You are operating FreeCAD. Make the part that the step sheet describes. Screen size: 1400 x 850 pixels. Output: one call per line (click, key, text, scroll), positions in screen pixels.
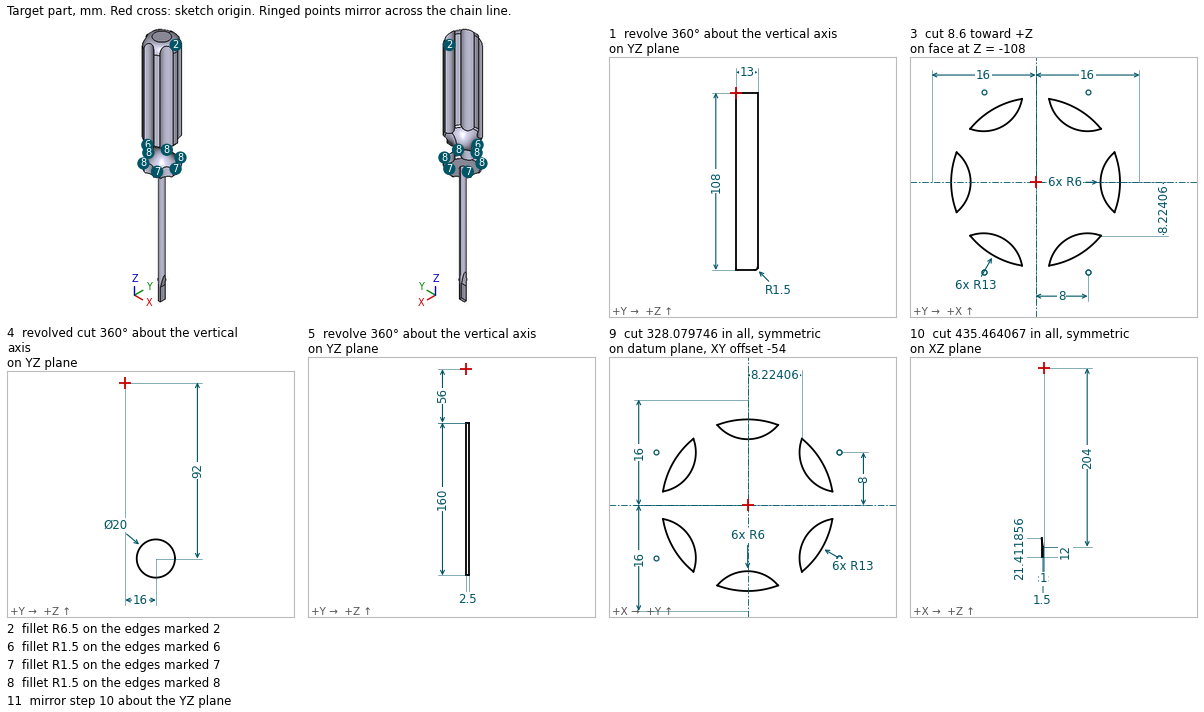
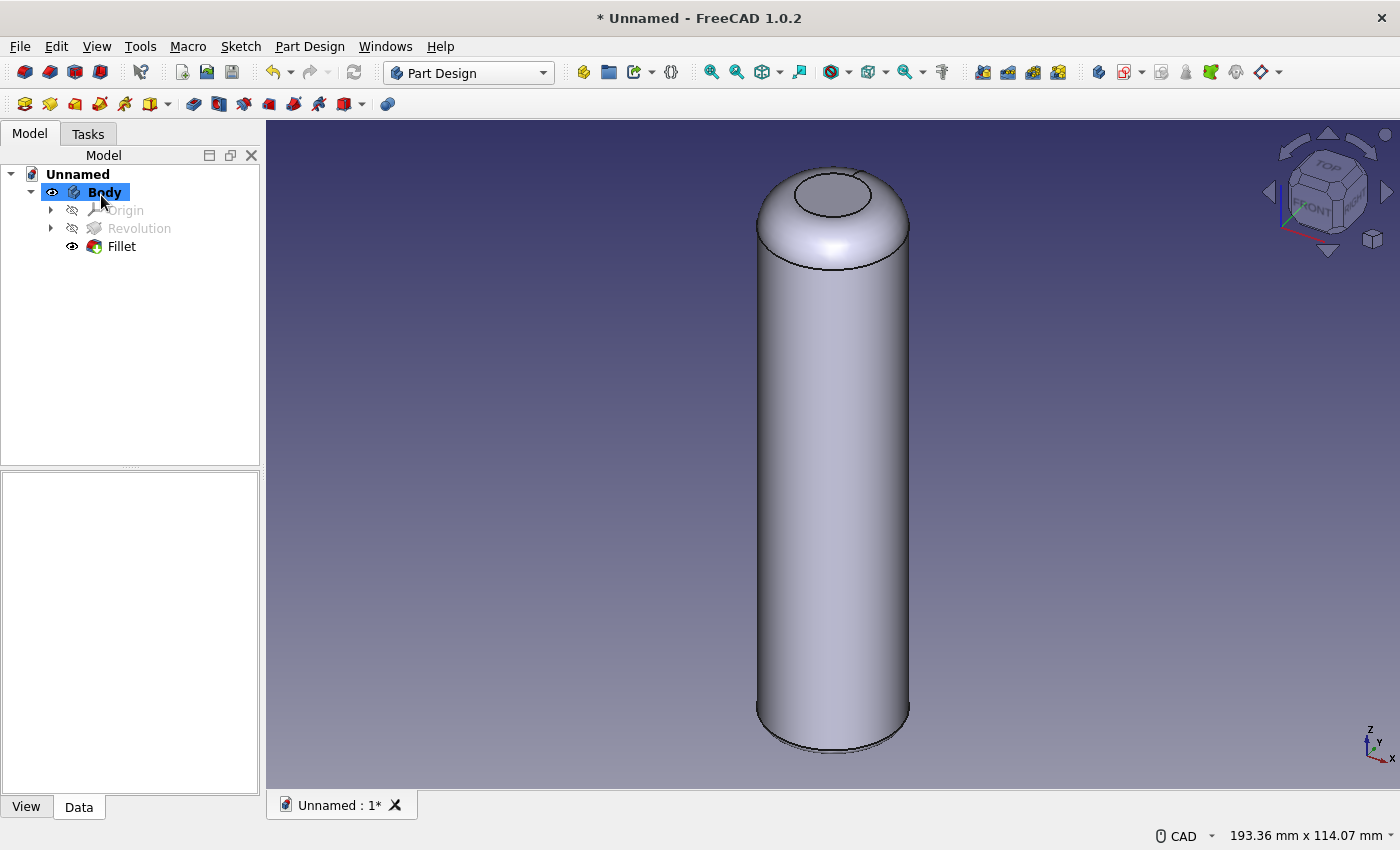
key(5)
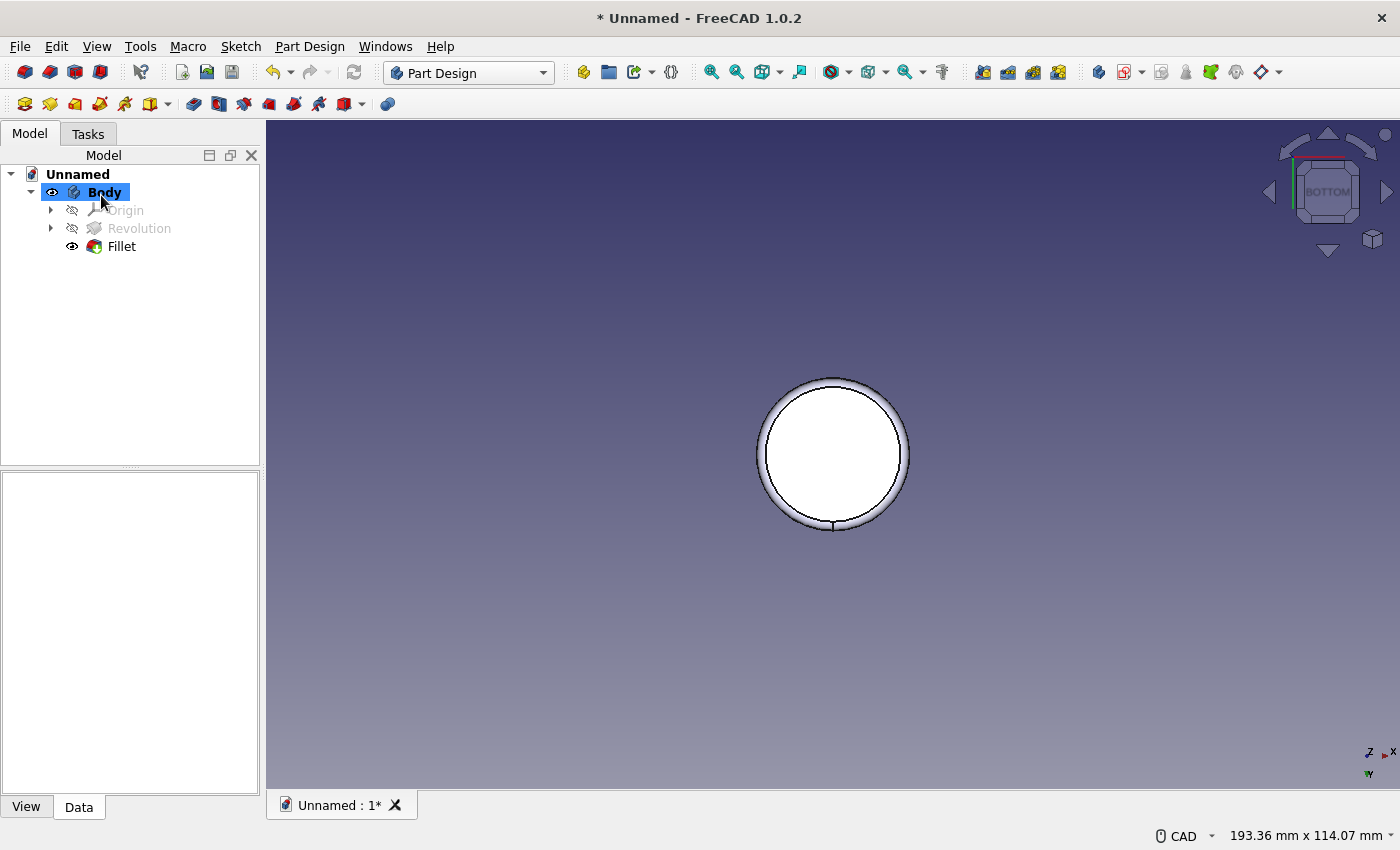
key(v)
key(f)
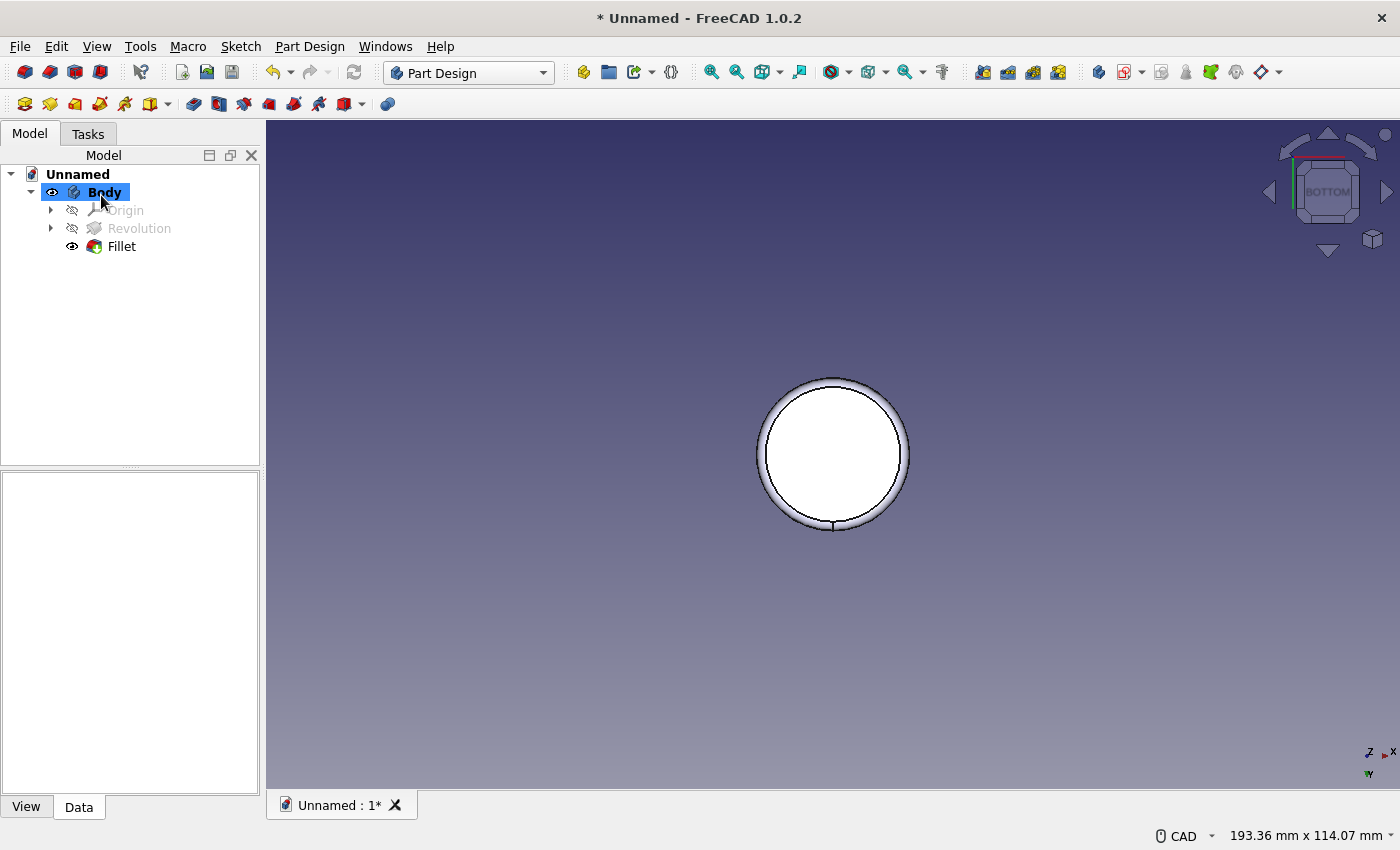
click(833, 453)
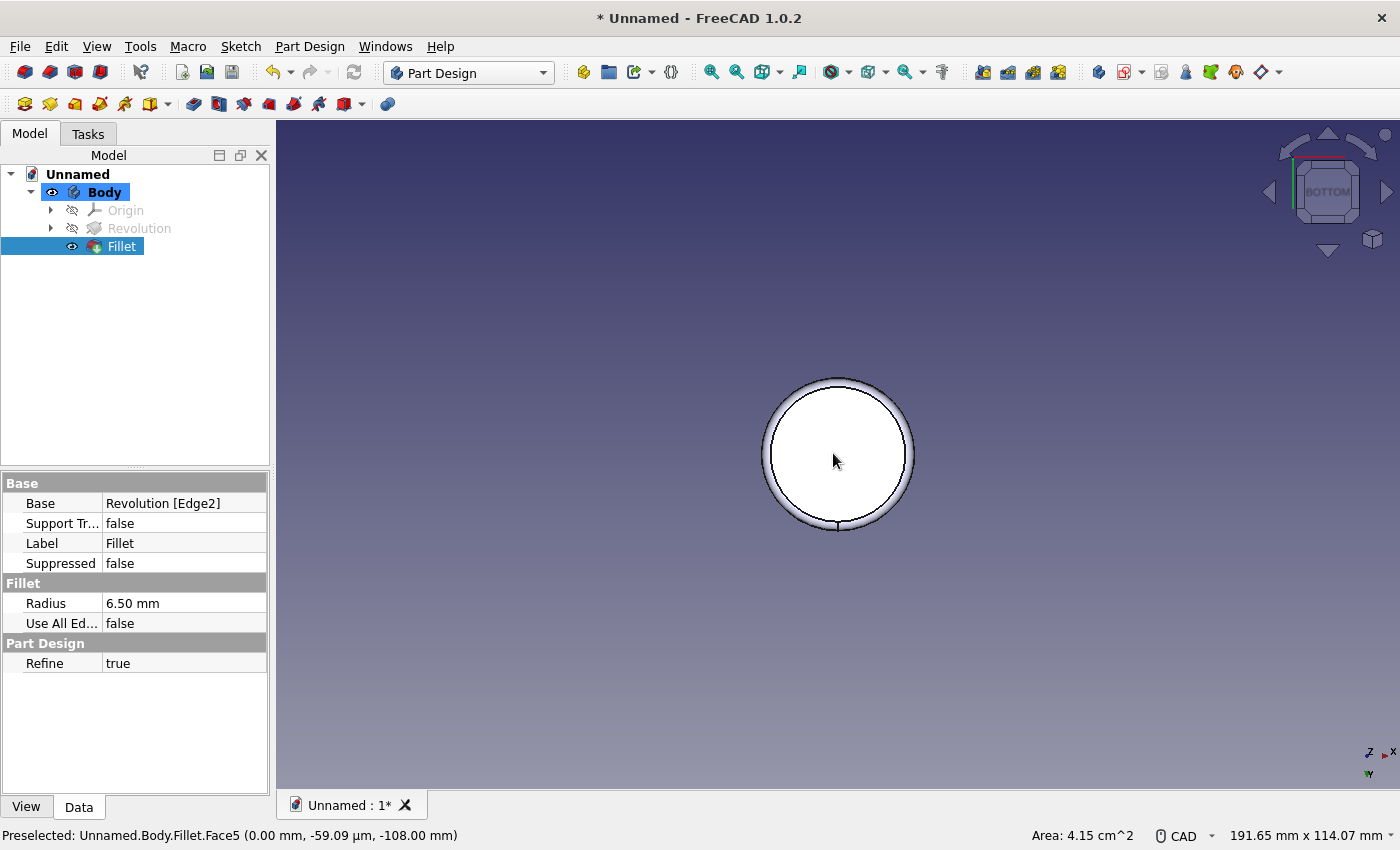
click(1124, 72)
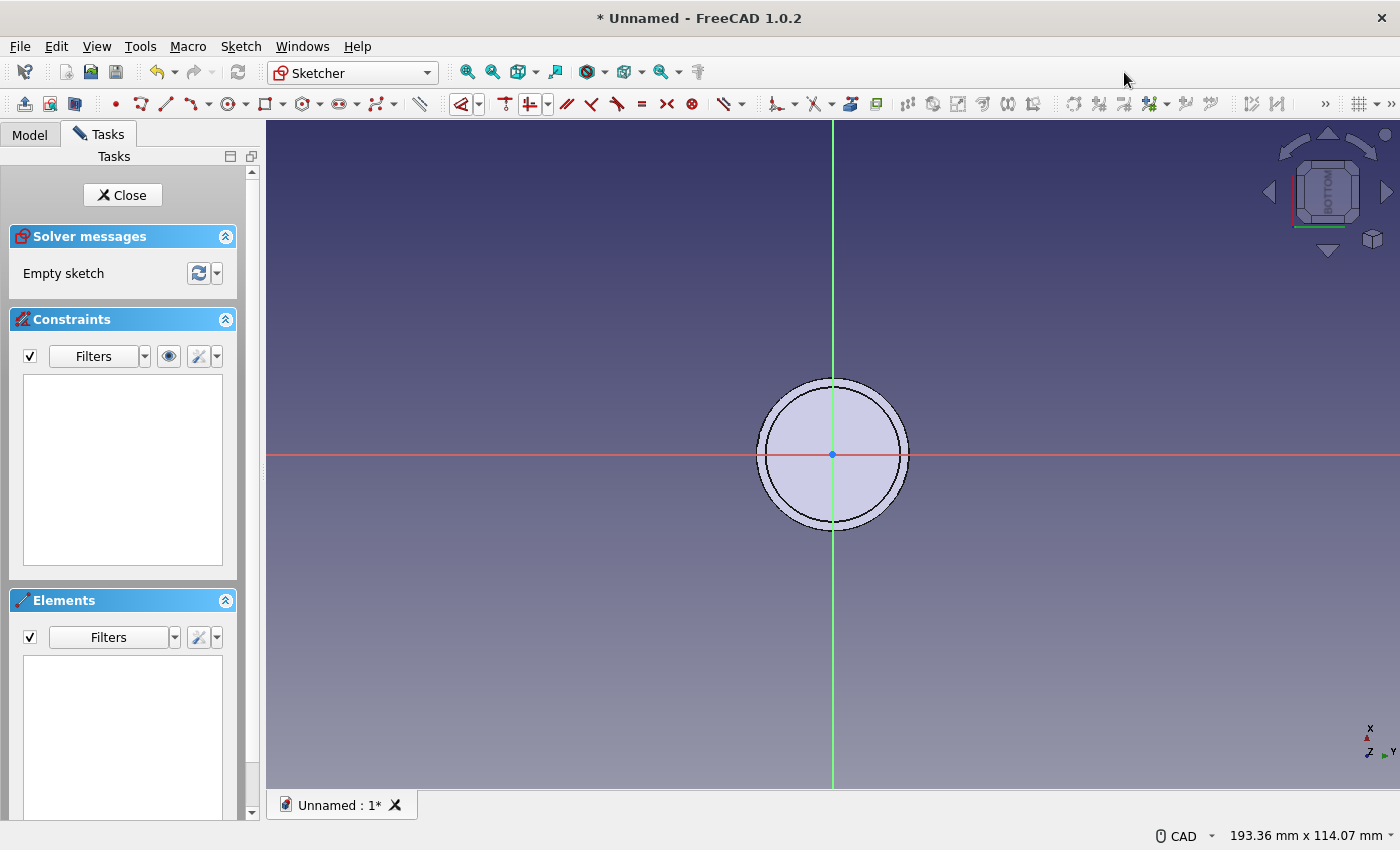
scroll(873, 454, up, 5)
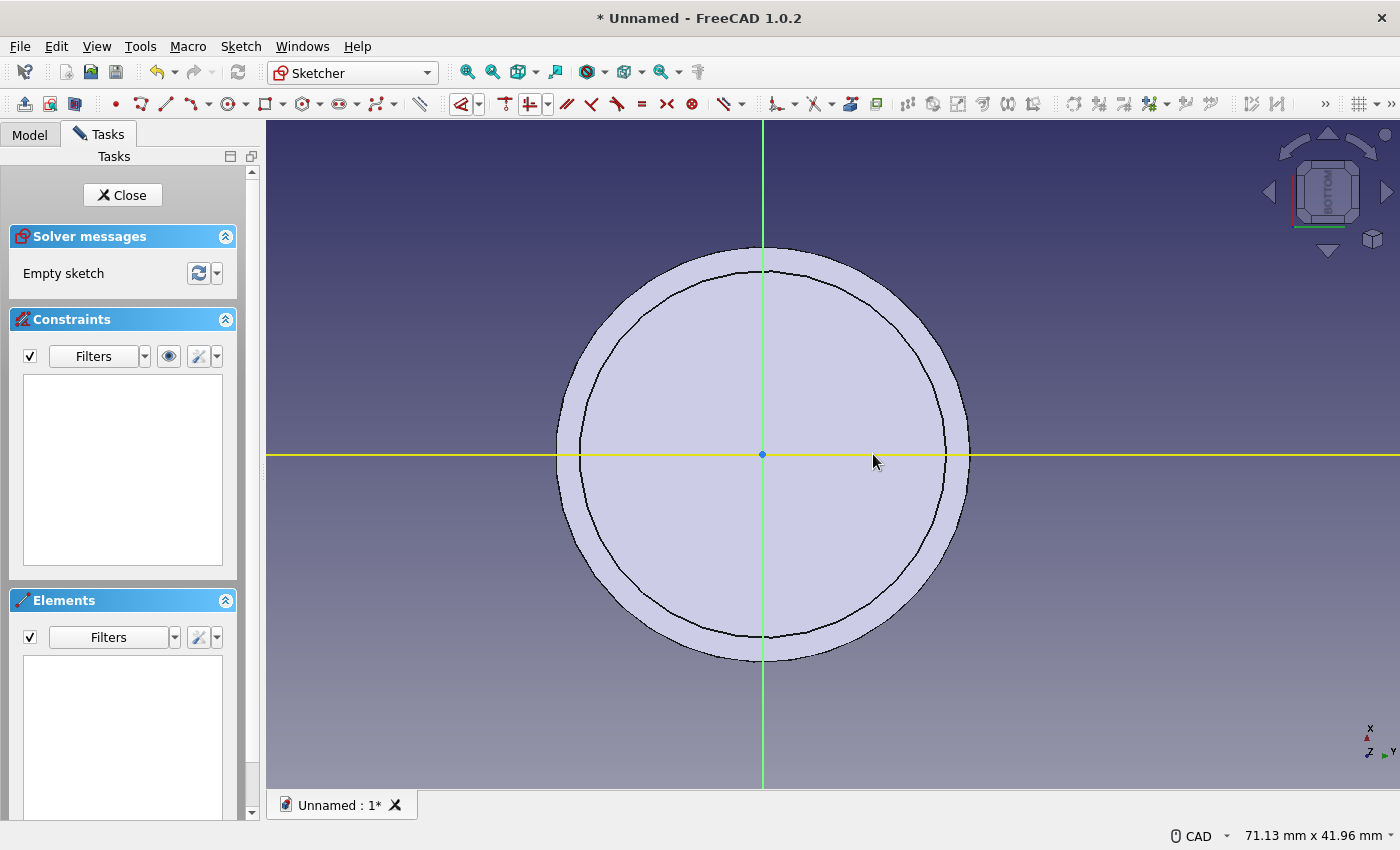
click(190, 104)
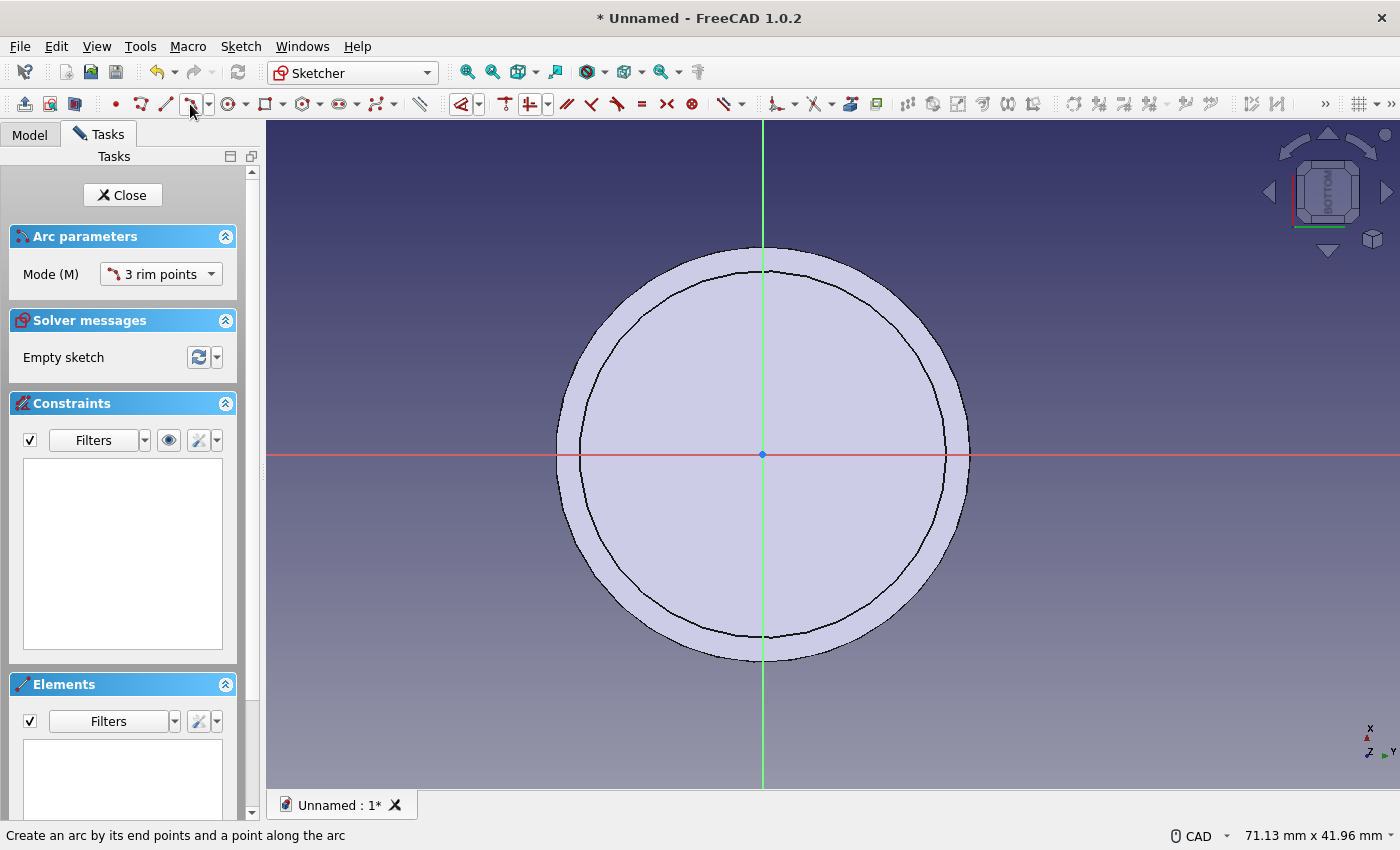
click(957, 381)
click(957, 528)
click(924, 438)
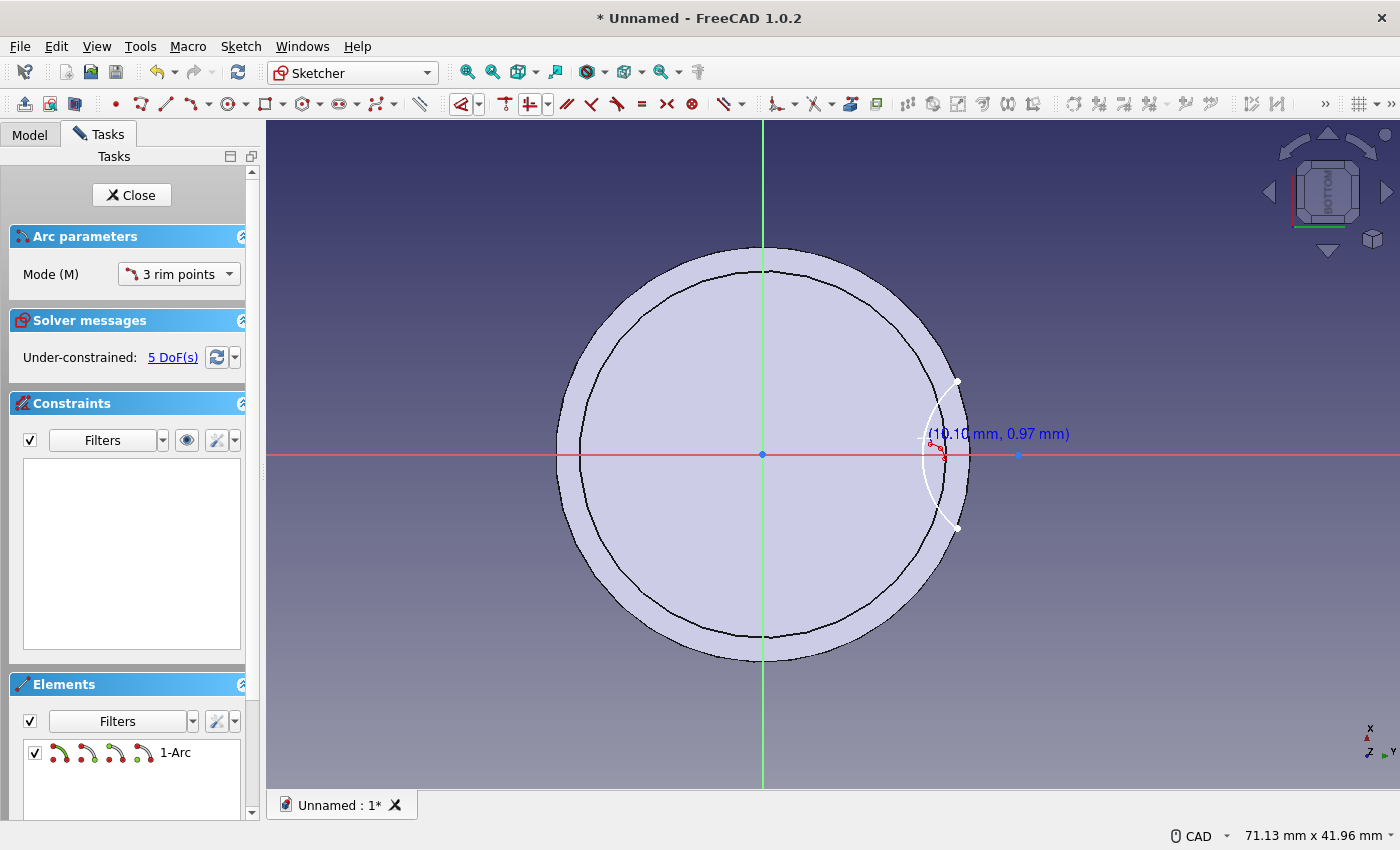
click(957, 529)
click(957, 382)